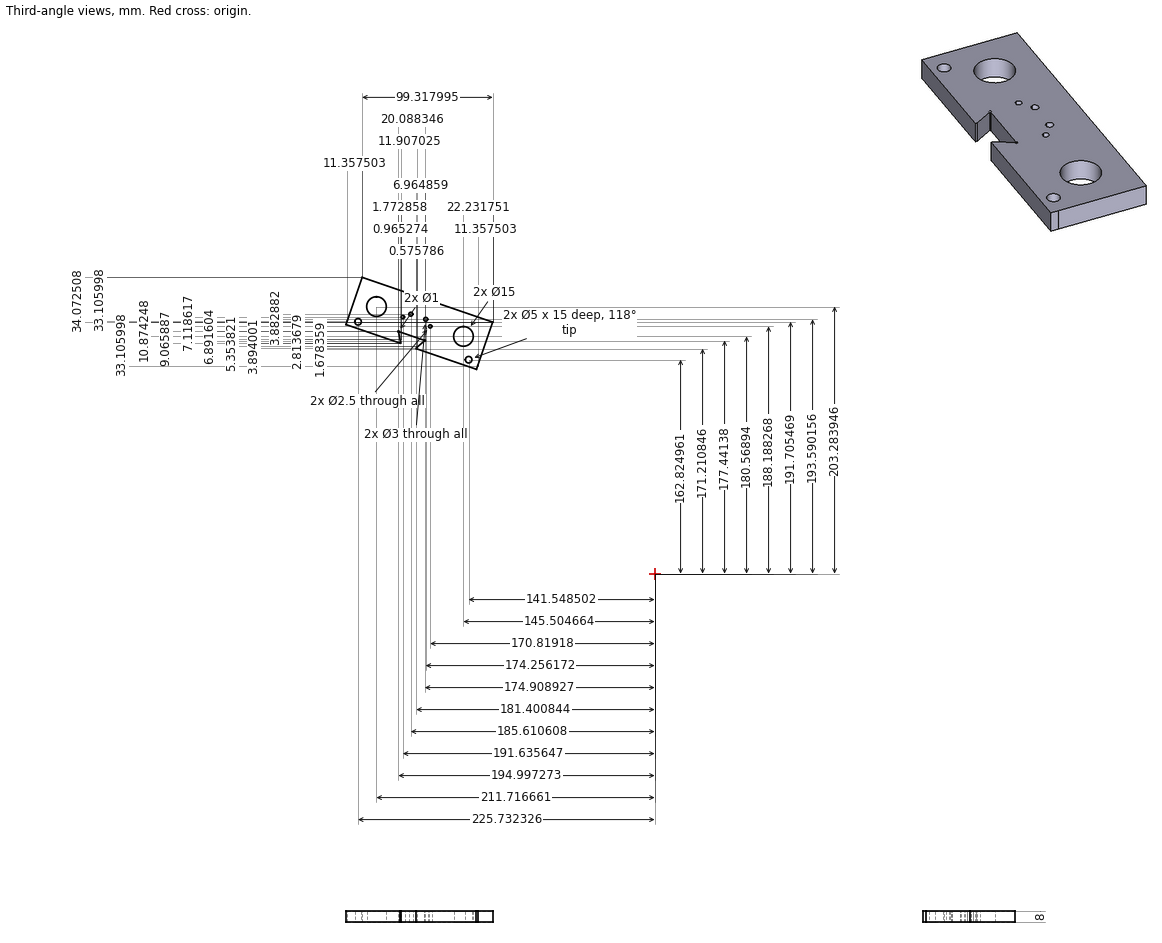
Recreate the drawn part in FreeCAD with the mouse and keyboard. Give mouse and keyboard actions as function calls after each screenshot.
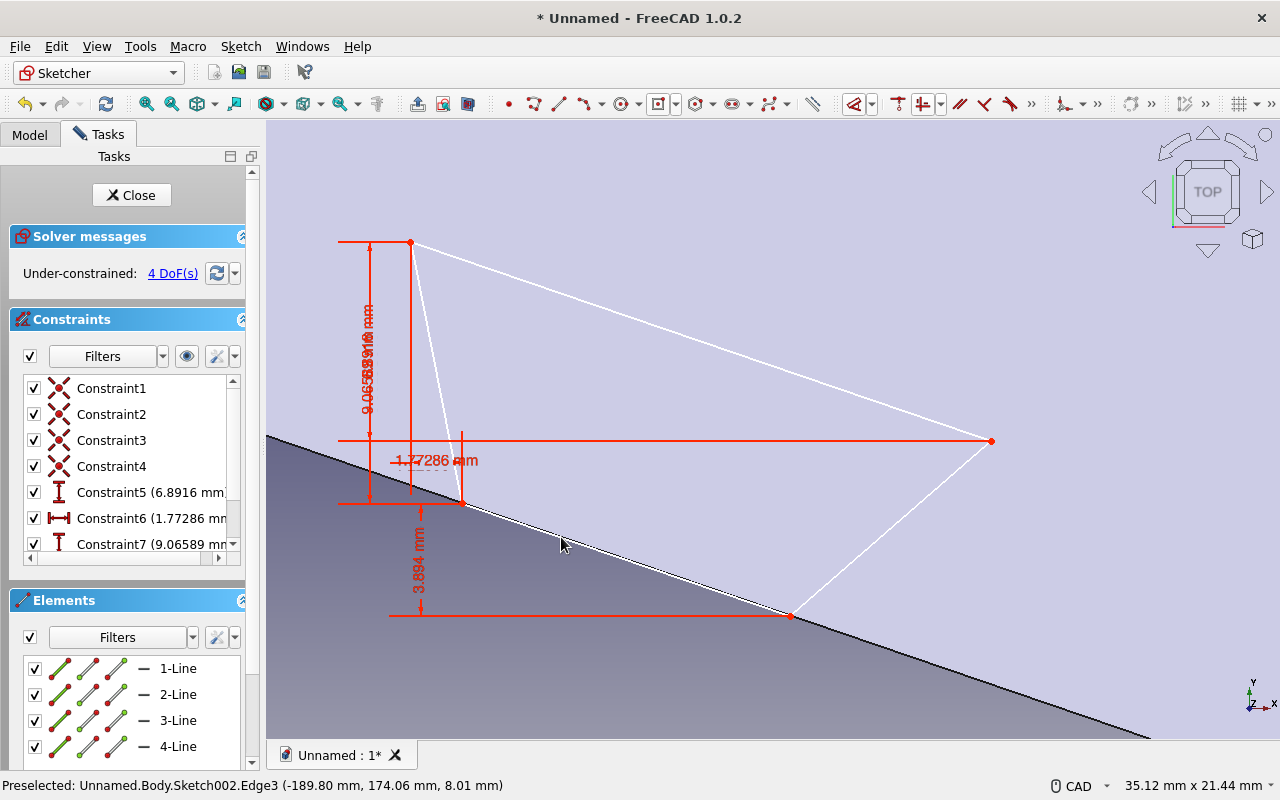
click(850, 564)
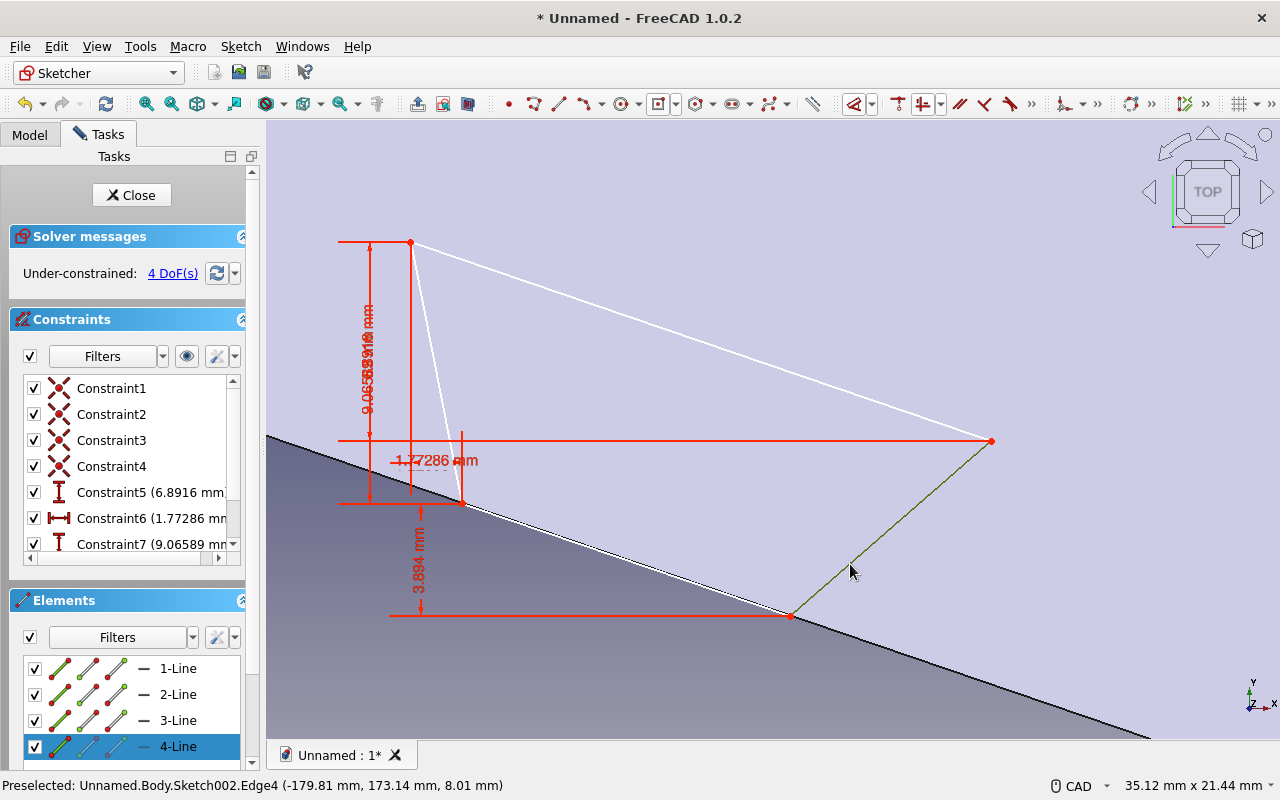
click(872, 104)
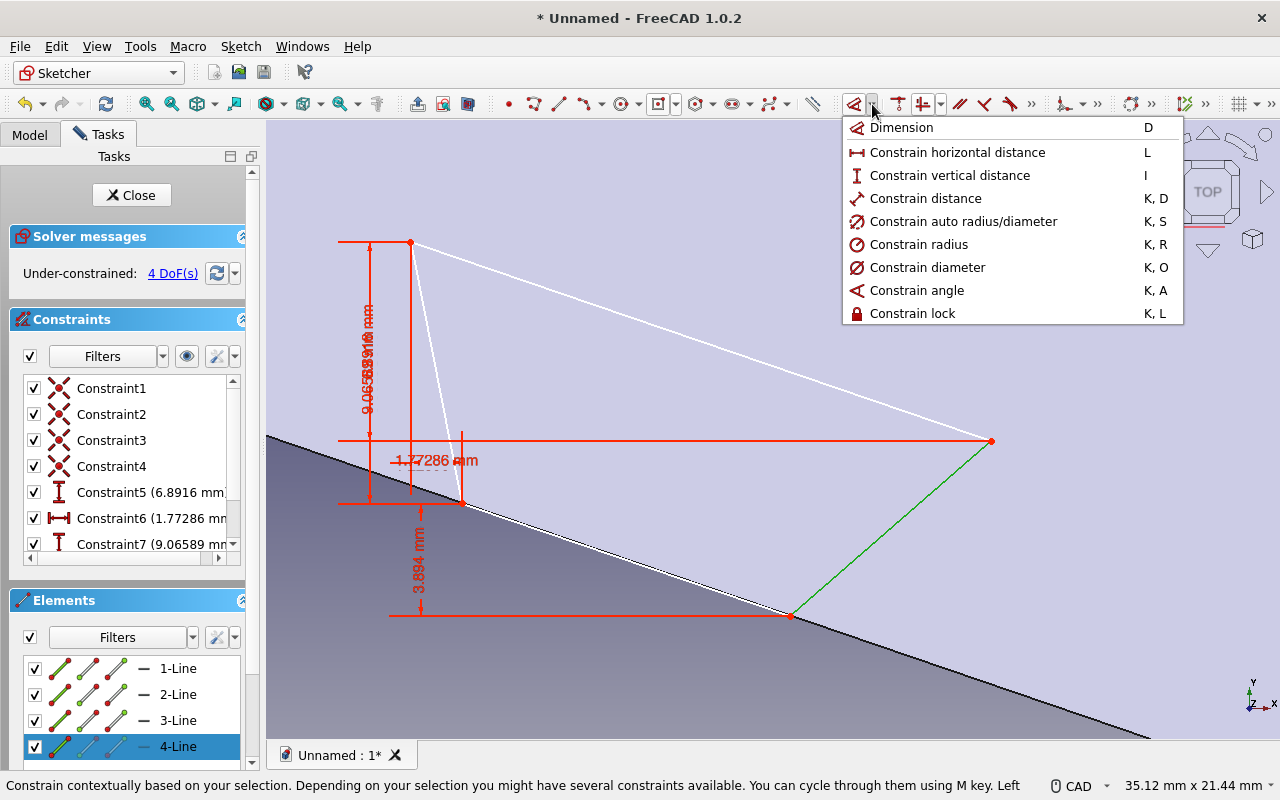
click(1013, 152)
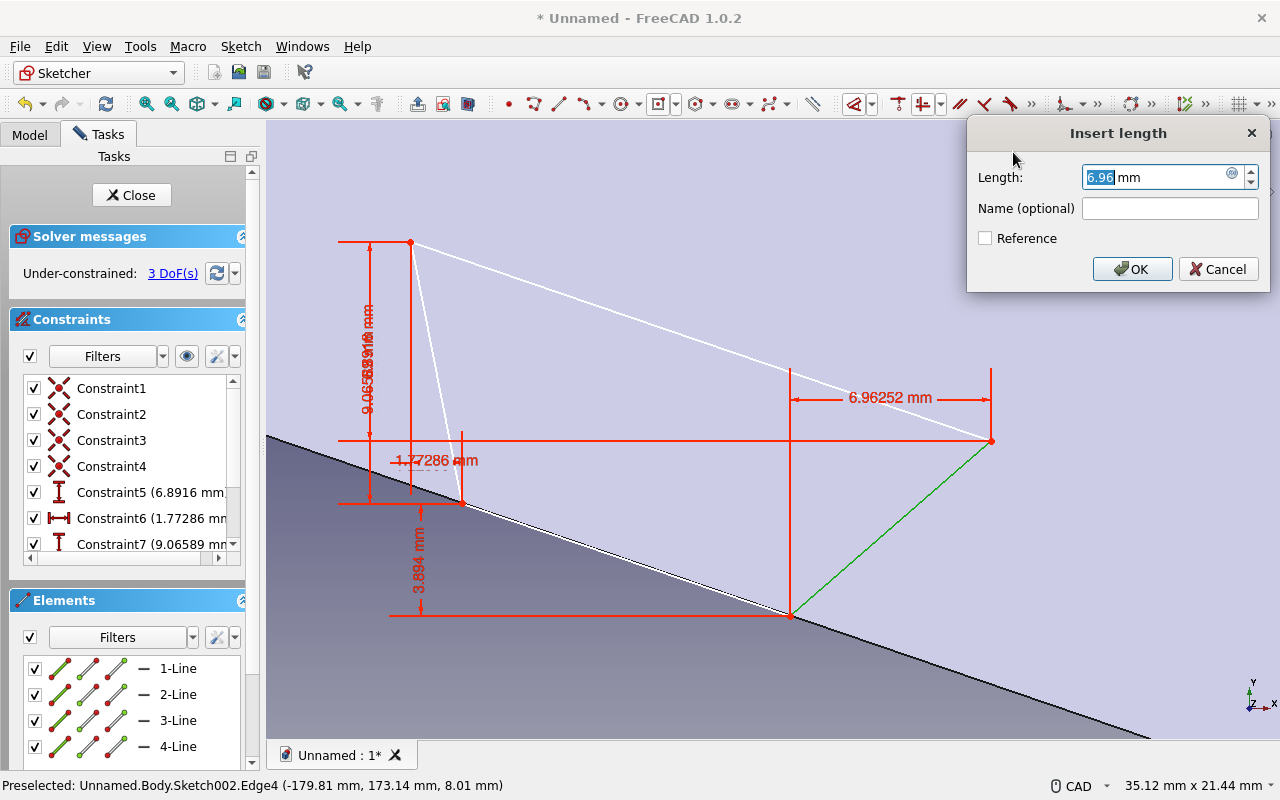
text(6.964859)
key(Return)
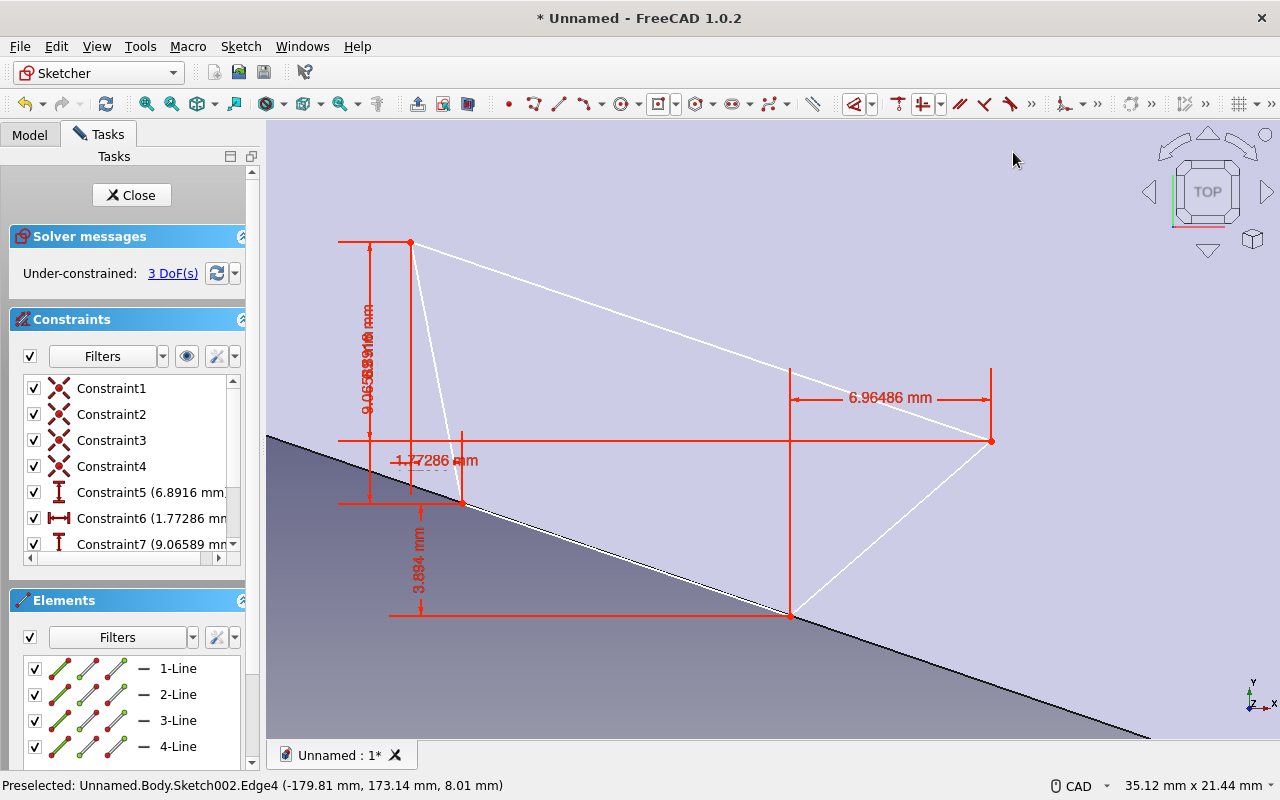
click(991, 441)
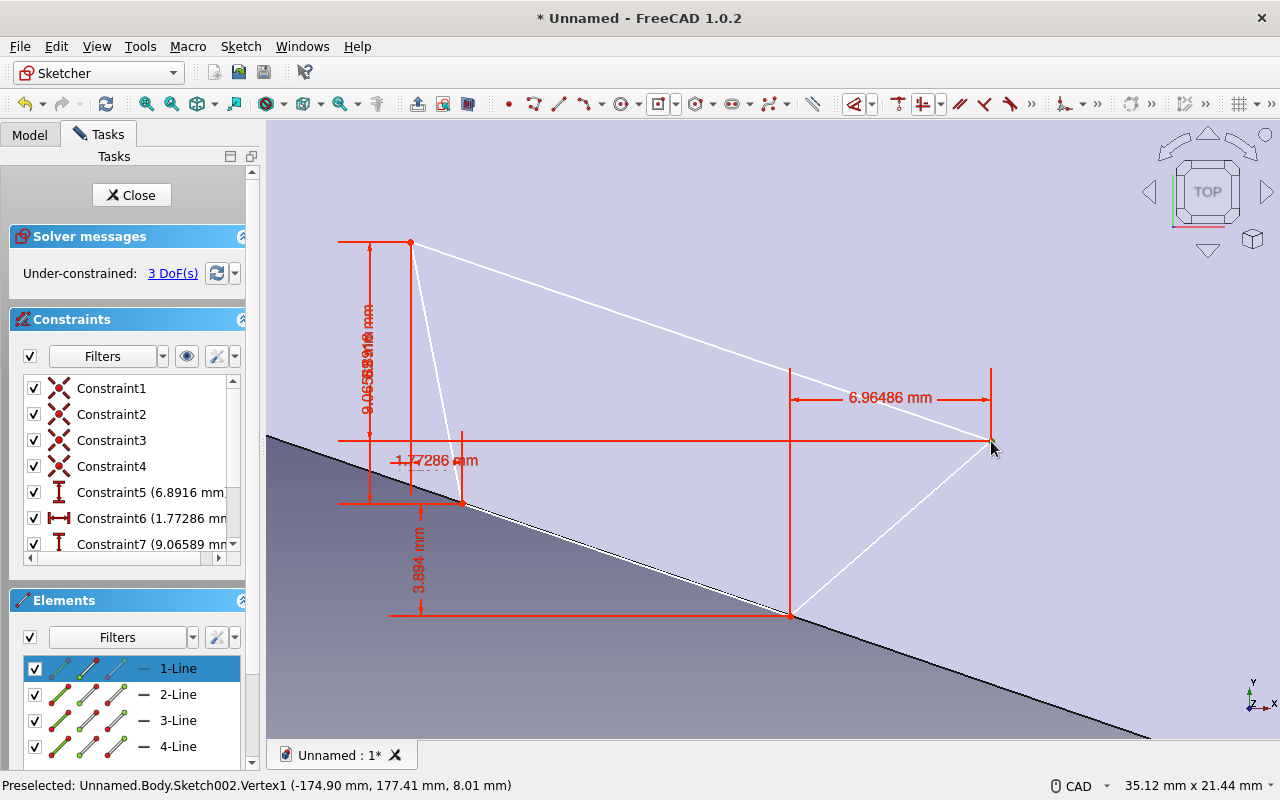
key(i)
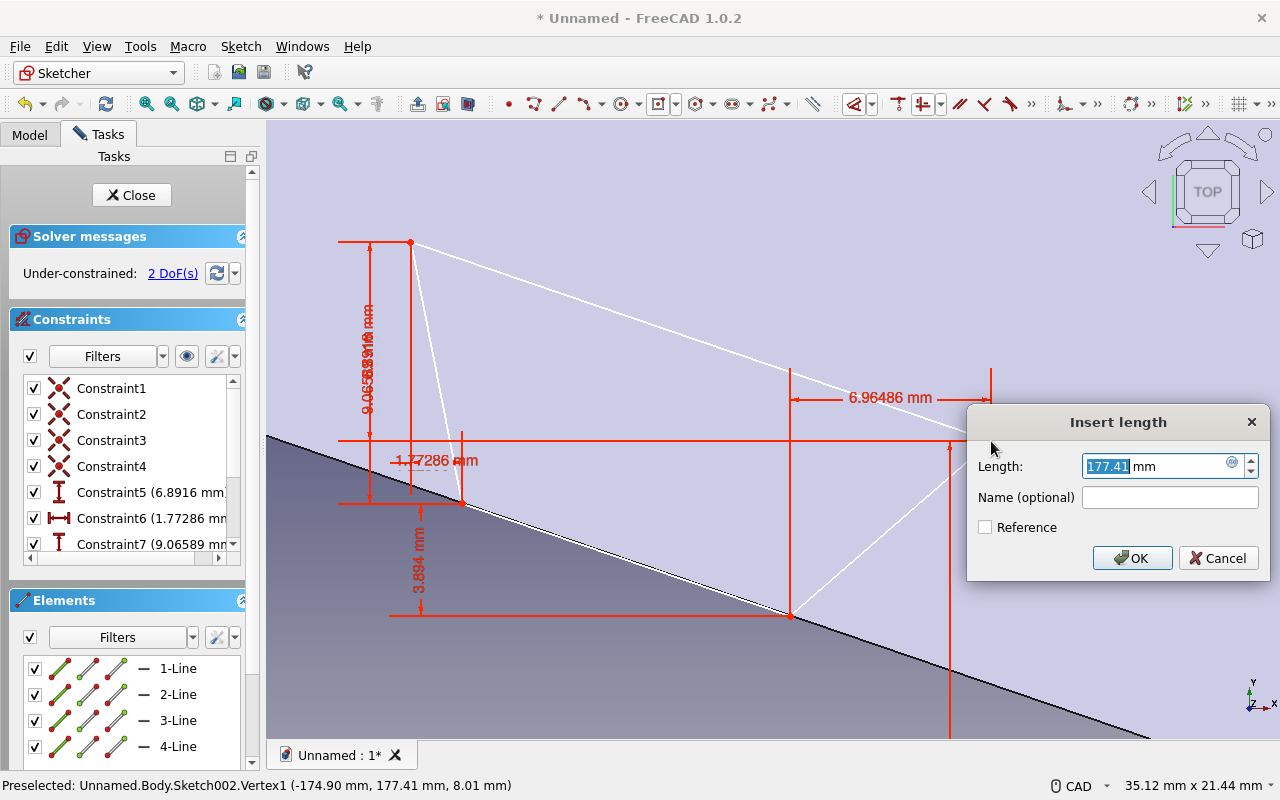
text(177.44138)
key(Return)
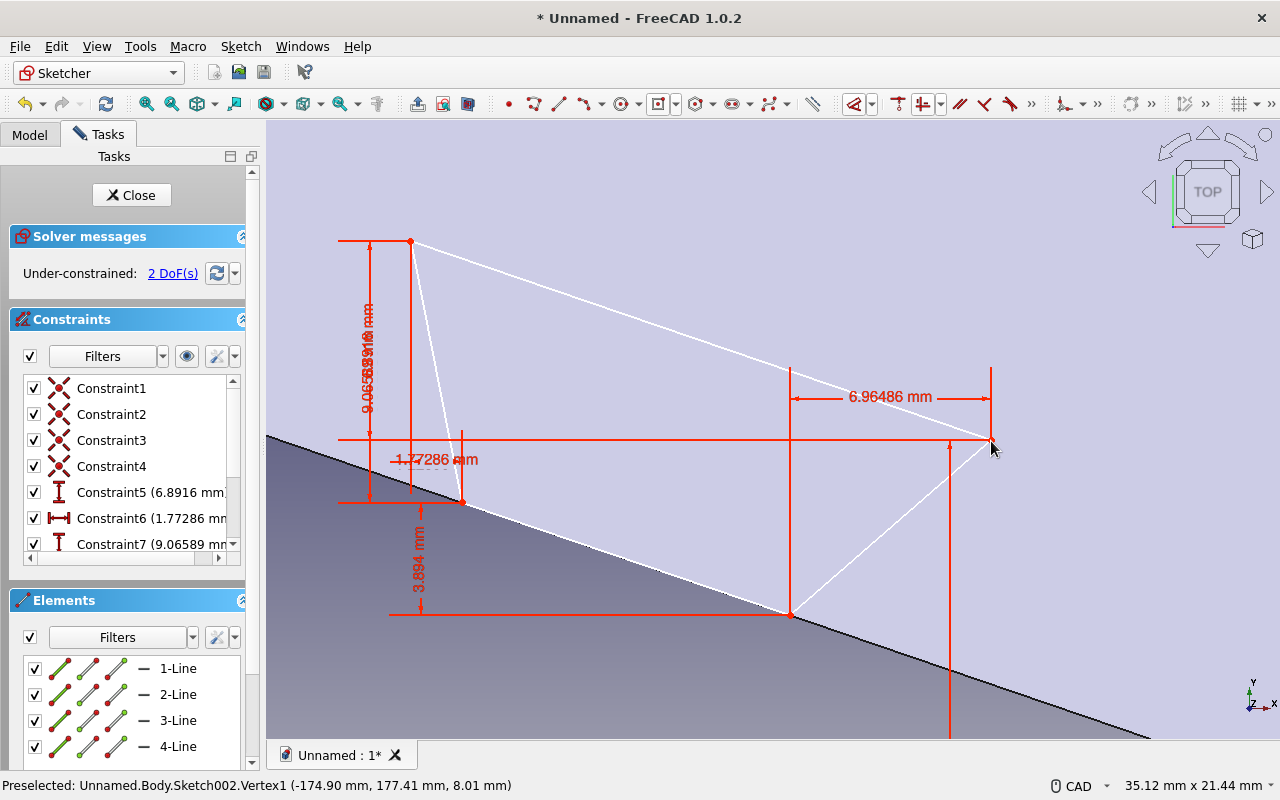
click(817, 380)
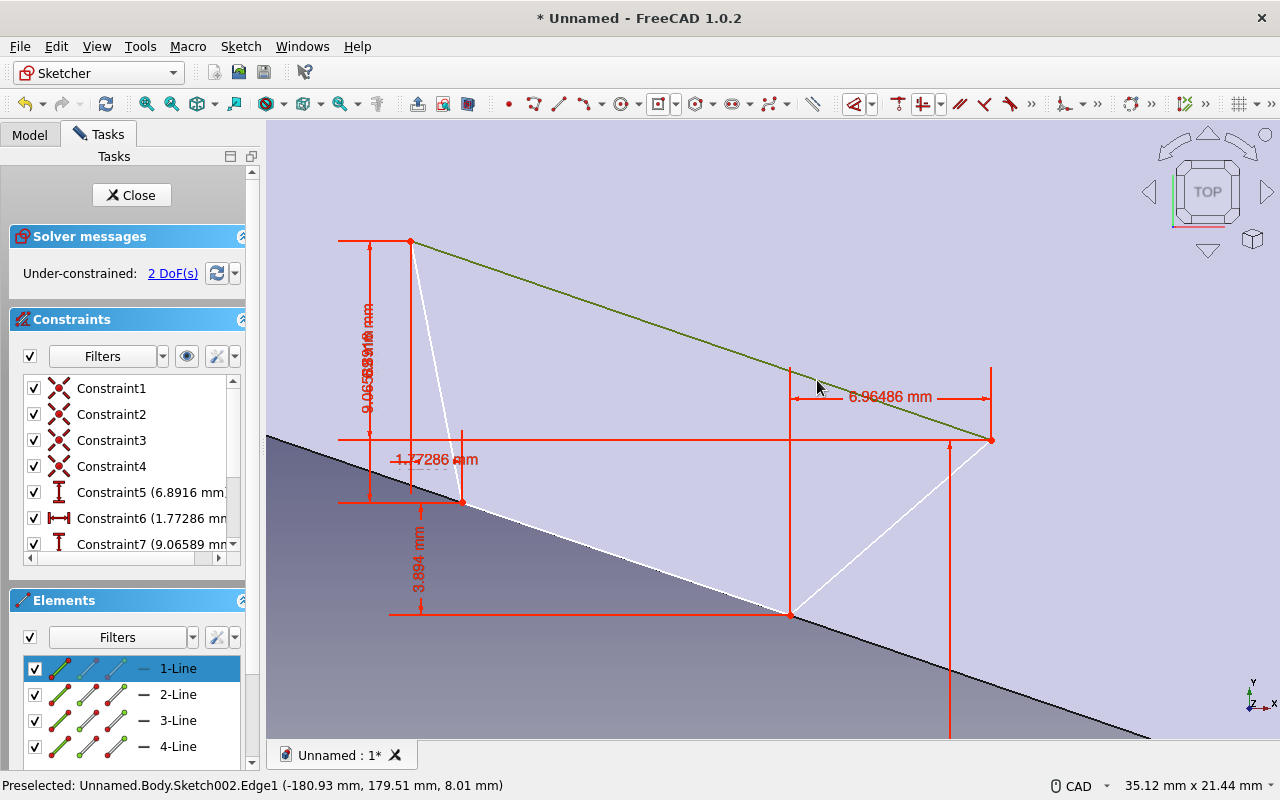
click(872, 104)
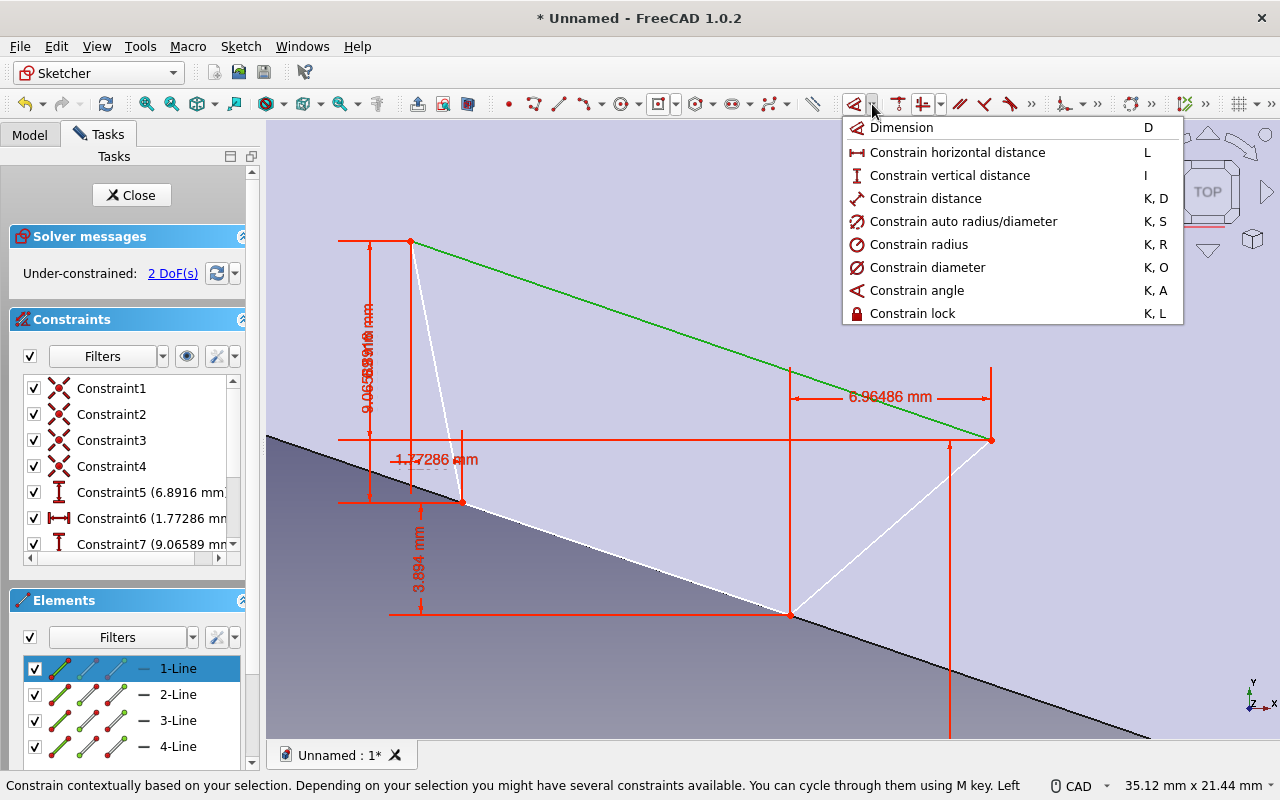
click(1013, 152)